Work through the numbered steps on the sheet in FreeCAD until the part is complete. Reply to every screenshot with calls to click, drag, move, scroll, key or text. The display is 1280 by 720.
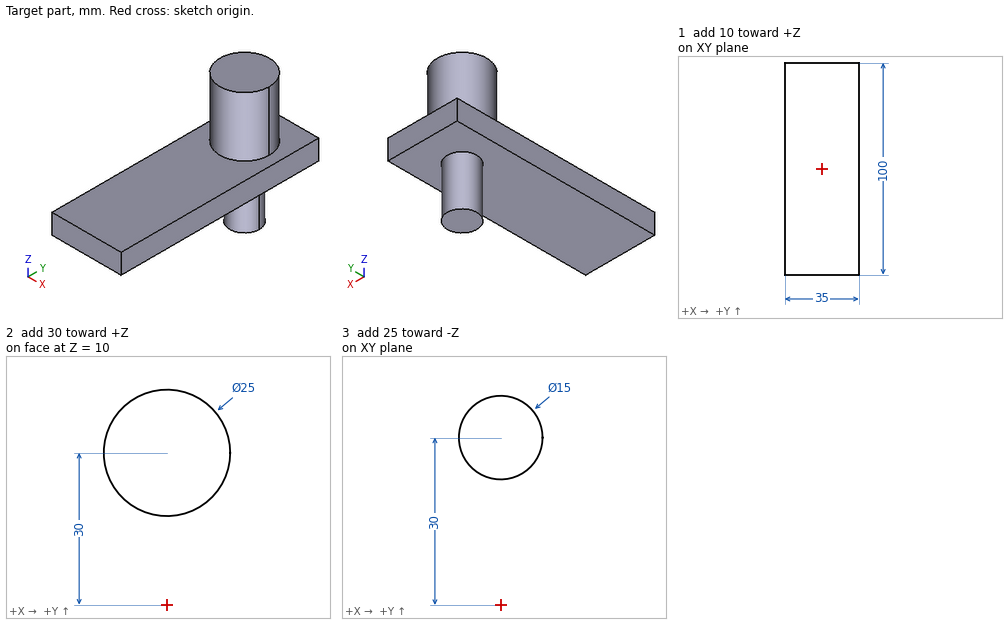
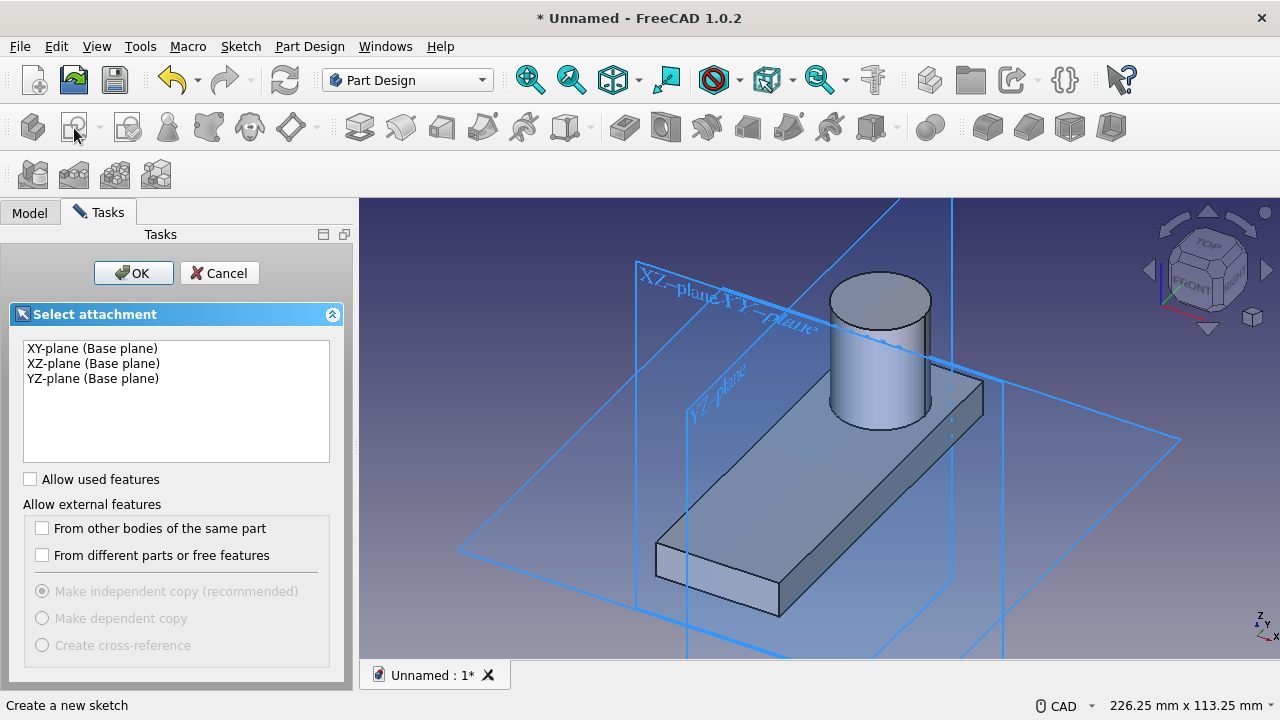
click(84, 348)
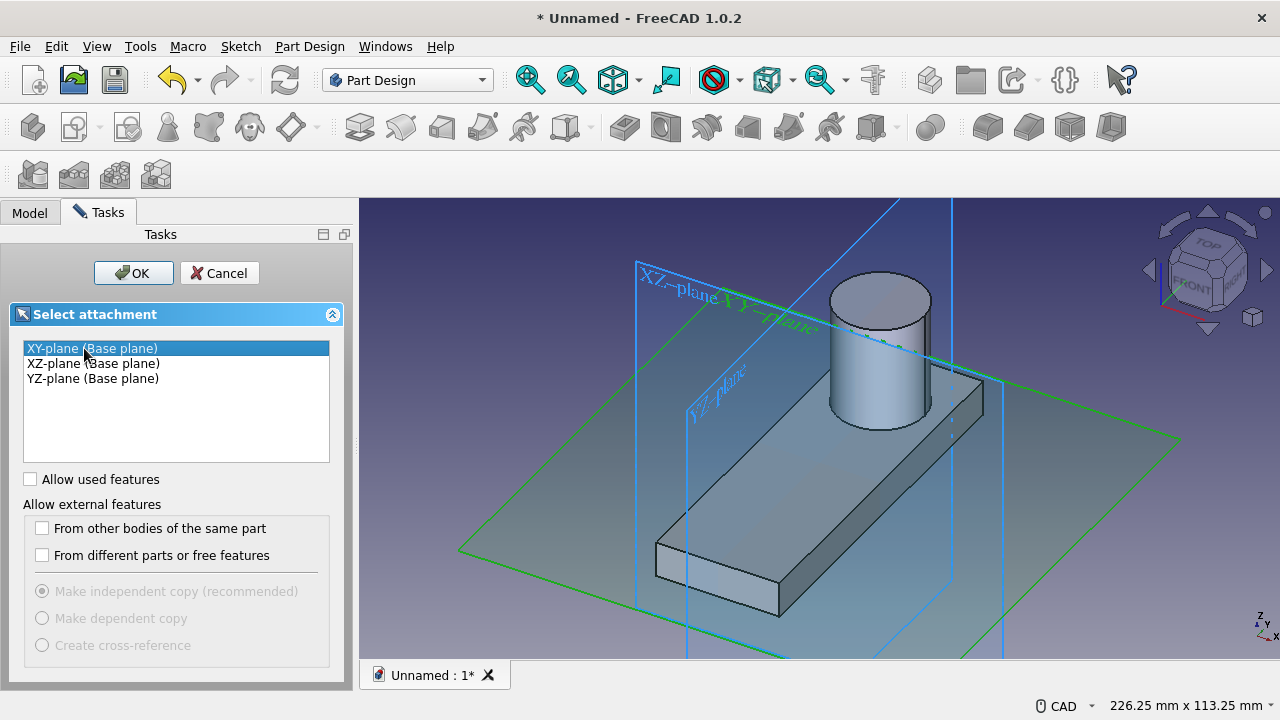
click(134, 273)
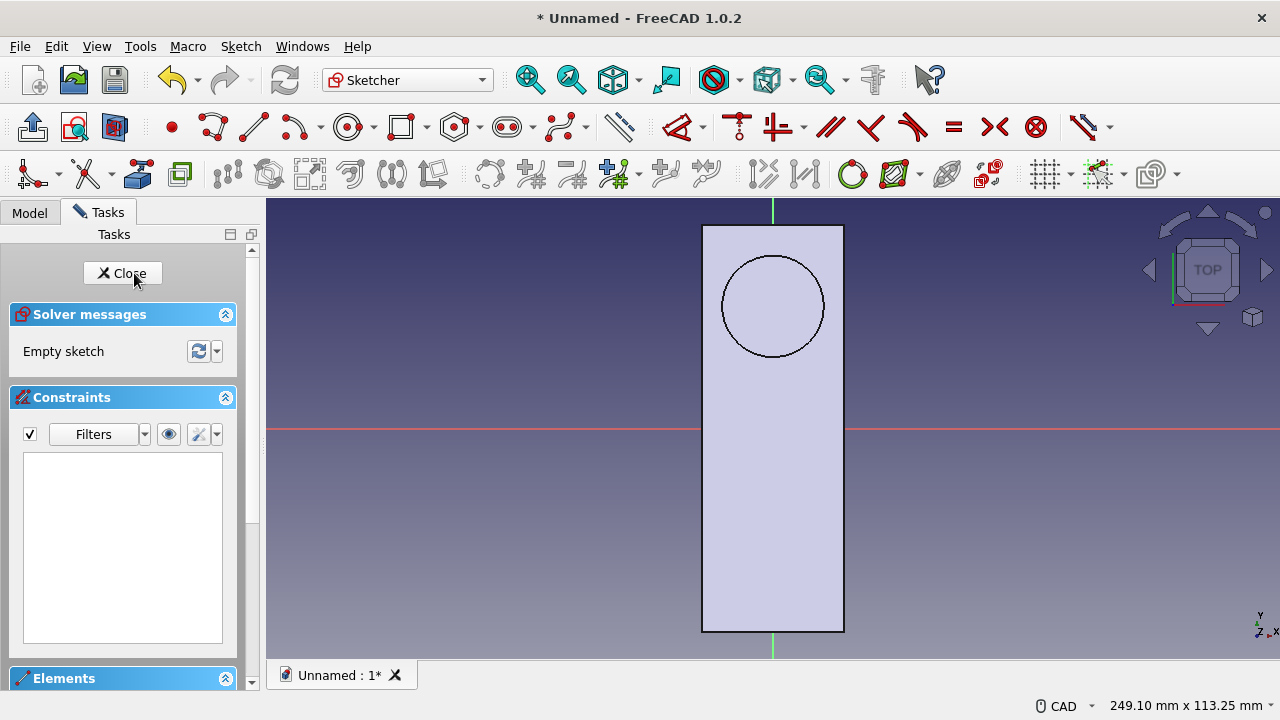
key(q)
key(s)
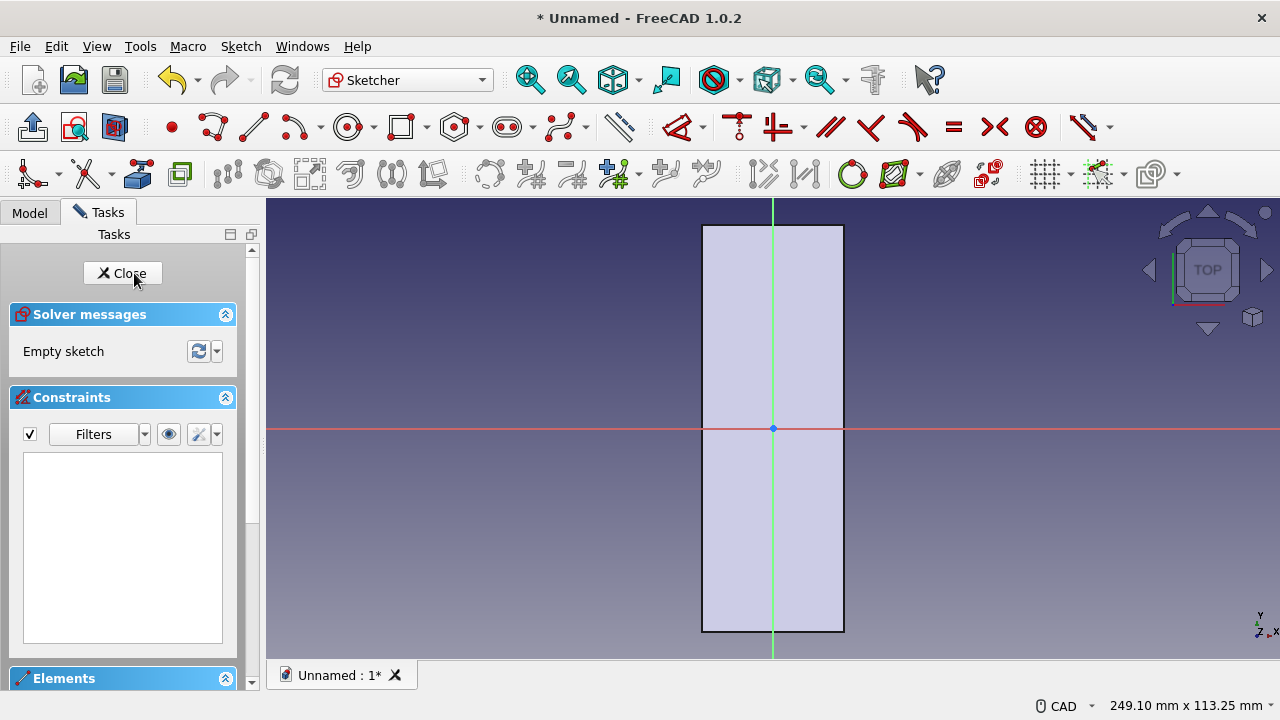
scroll(790, 275, up, 8)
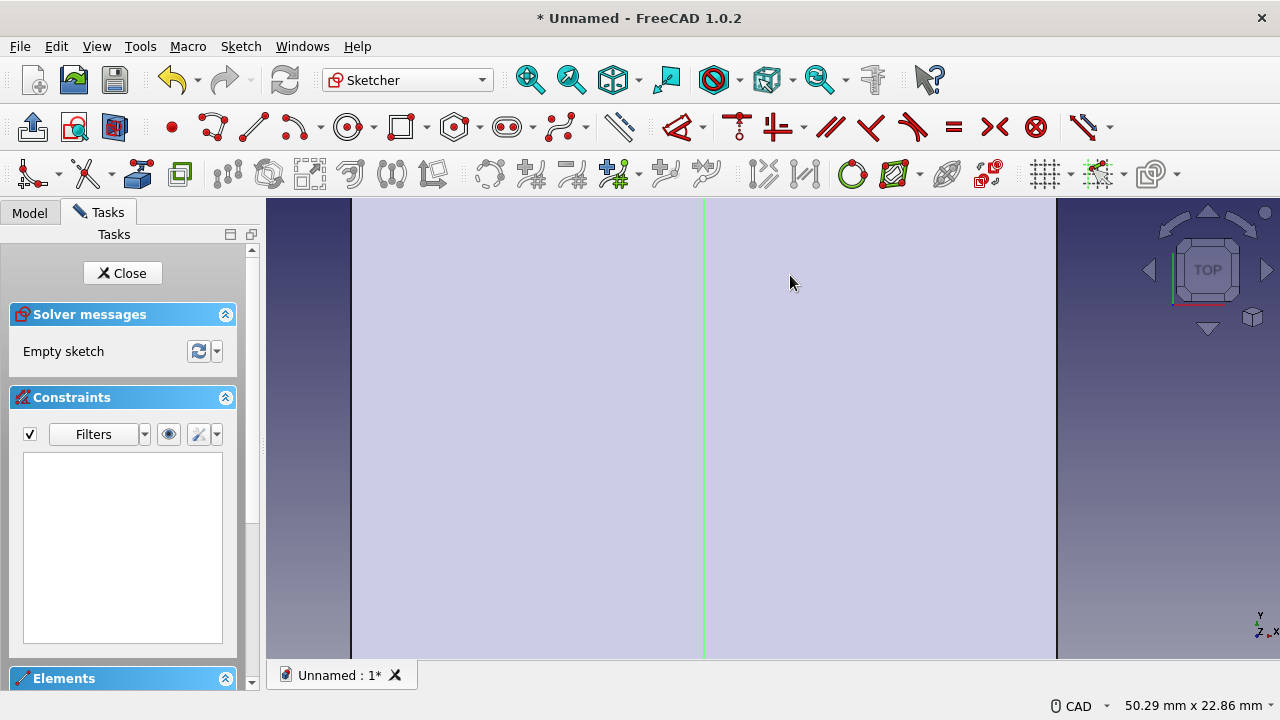
key(g)
key(c)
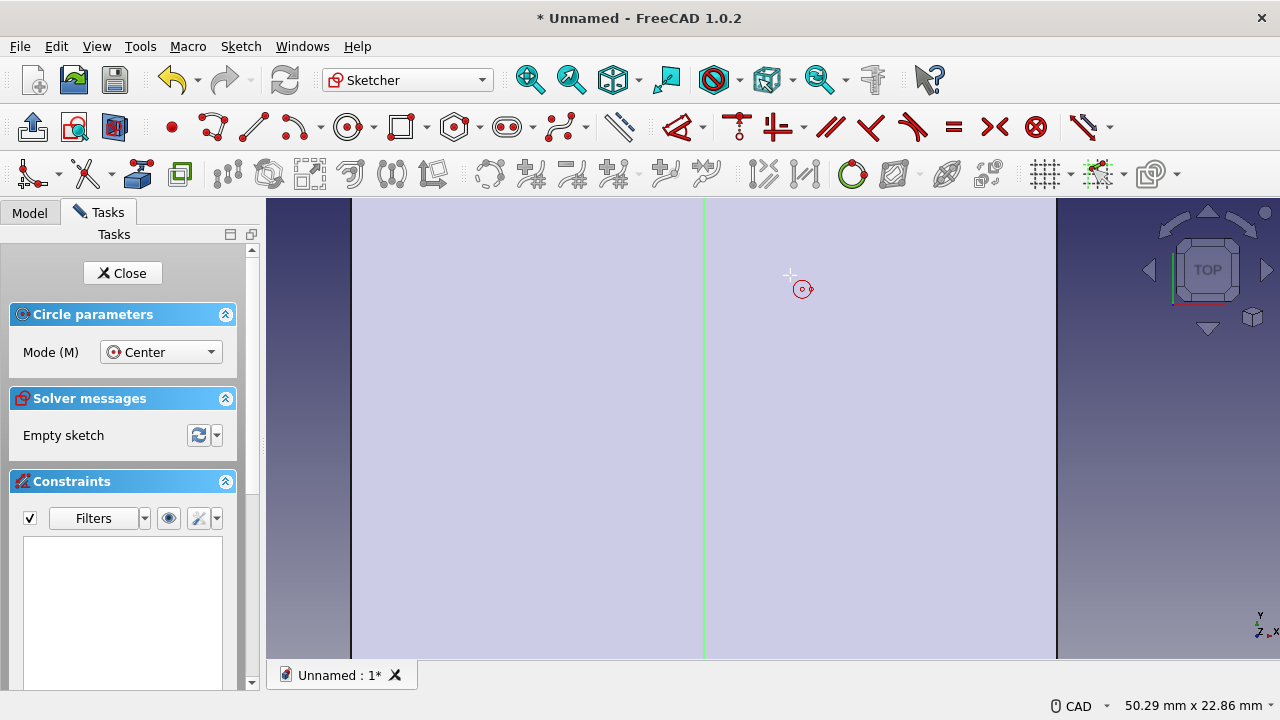
click(704, 430)
click(811, 323)
key(Escape)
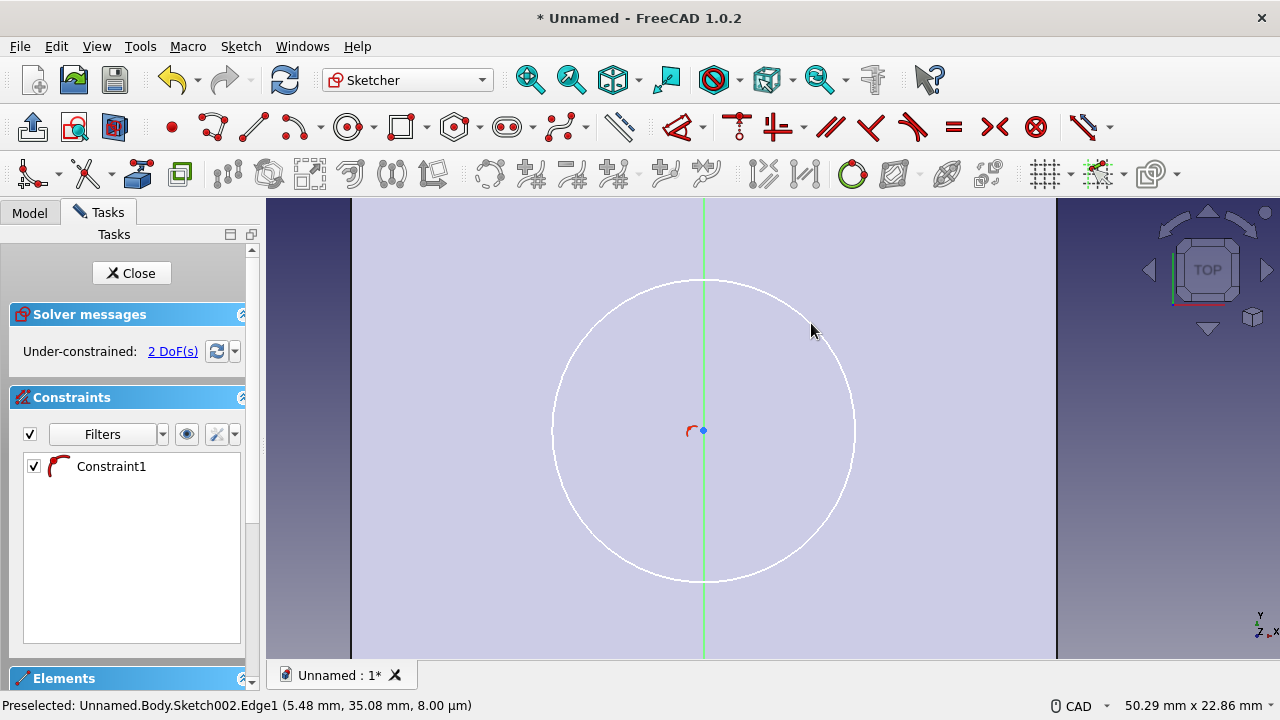
key(d)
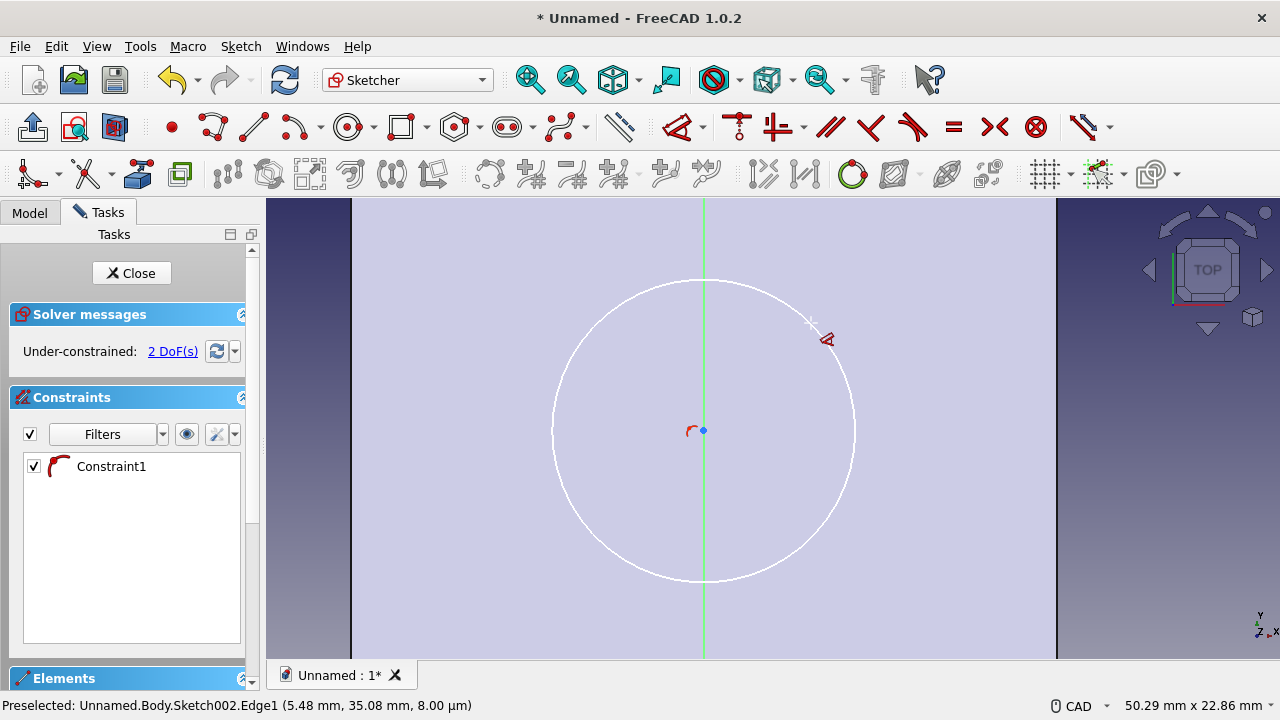
click(811, 324)
click(834, 301)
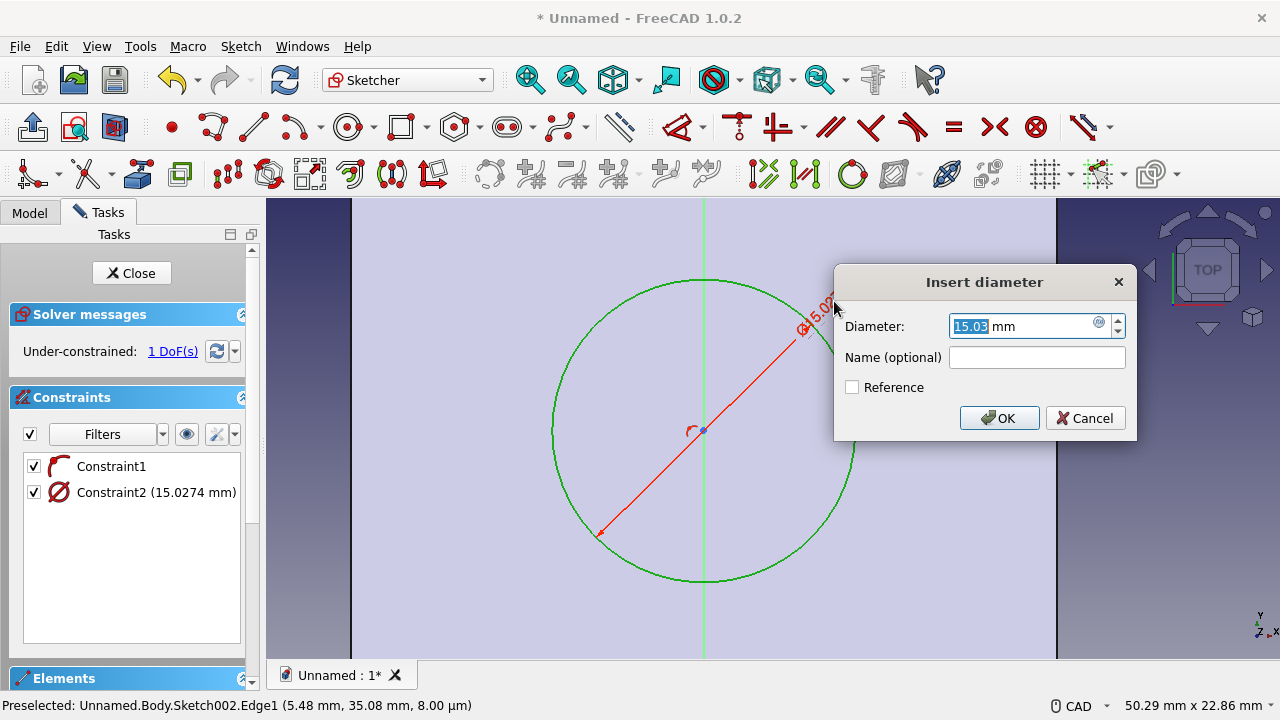
text(15)
key(Return)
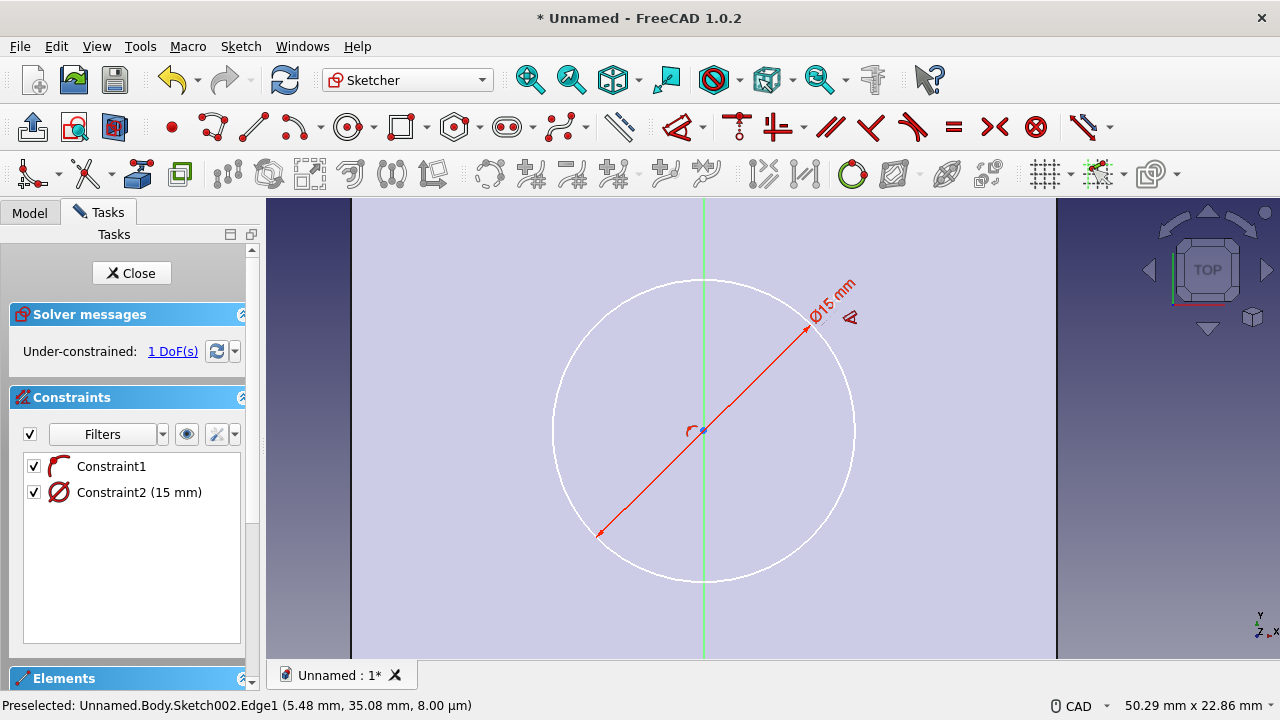
click(704, 431)
click(738, 531)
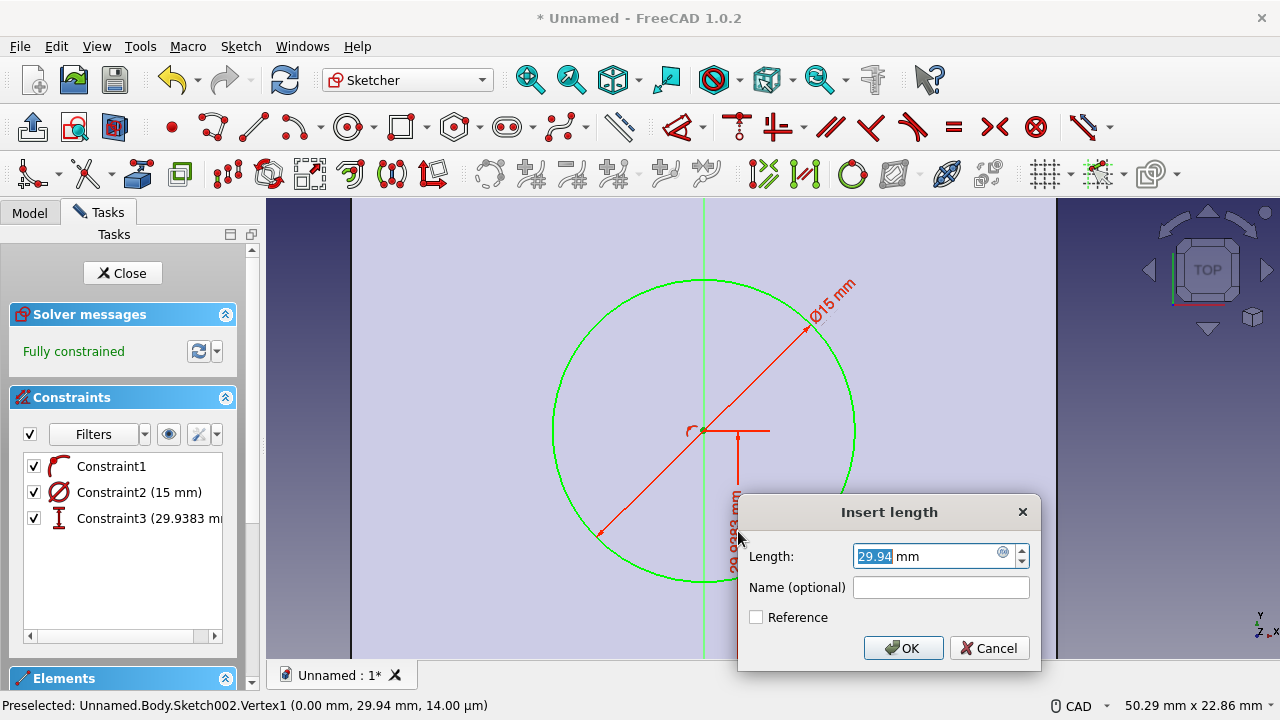
text(30)
key(Return)
key(Escape)